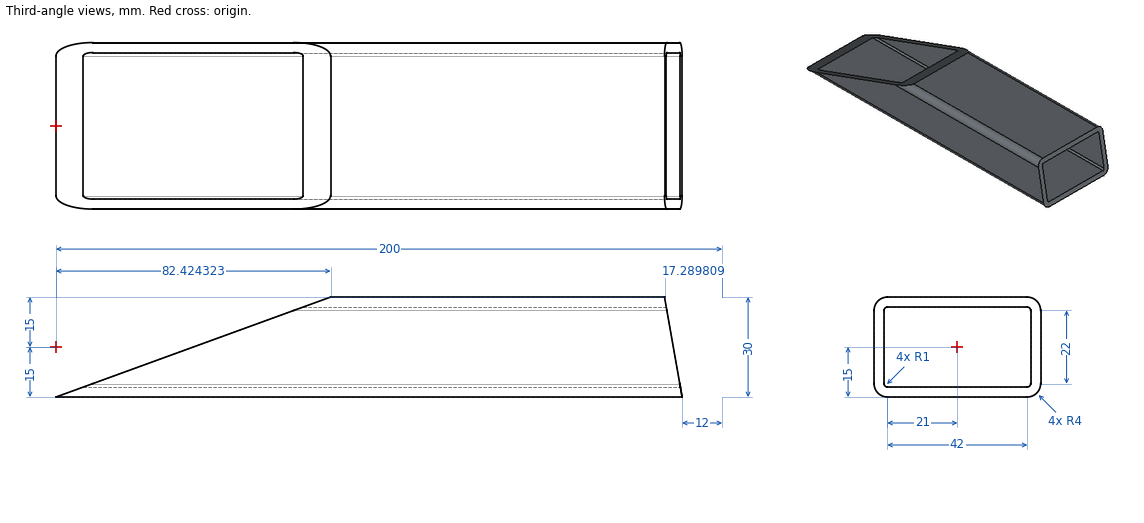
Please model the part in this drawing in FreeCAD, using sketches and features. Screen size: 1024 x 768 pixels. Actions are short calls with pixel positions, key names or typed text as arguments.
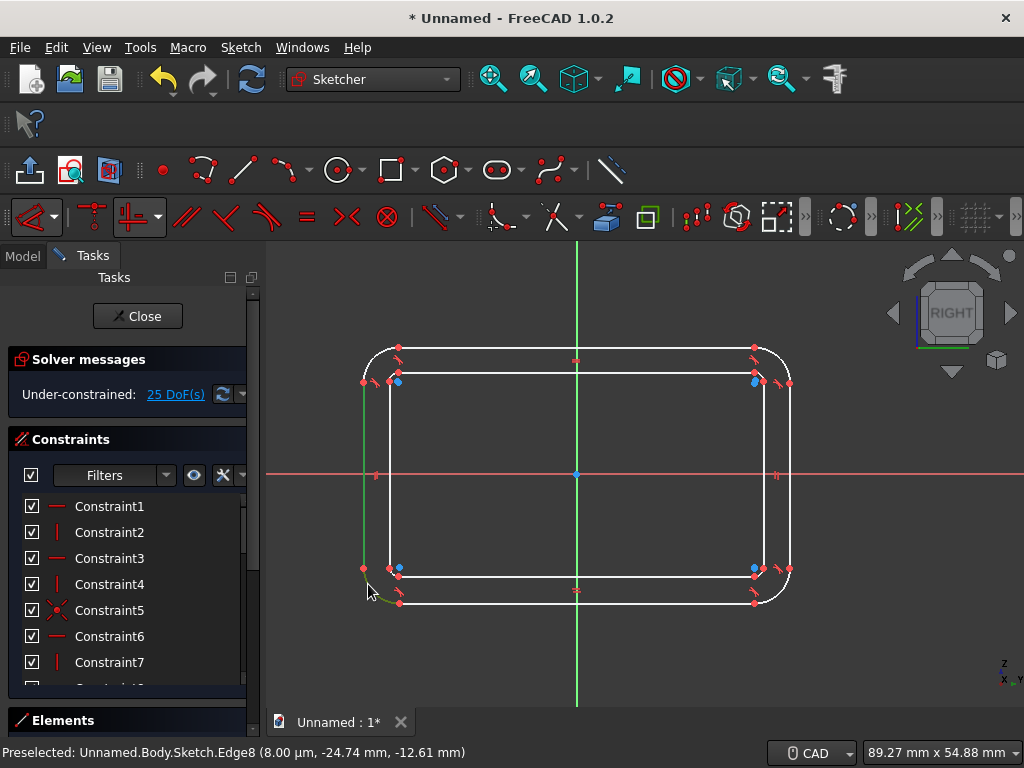
click(268, 218)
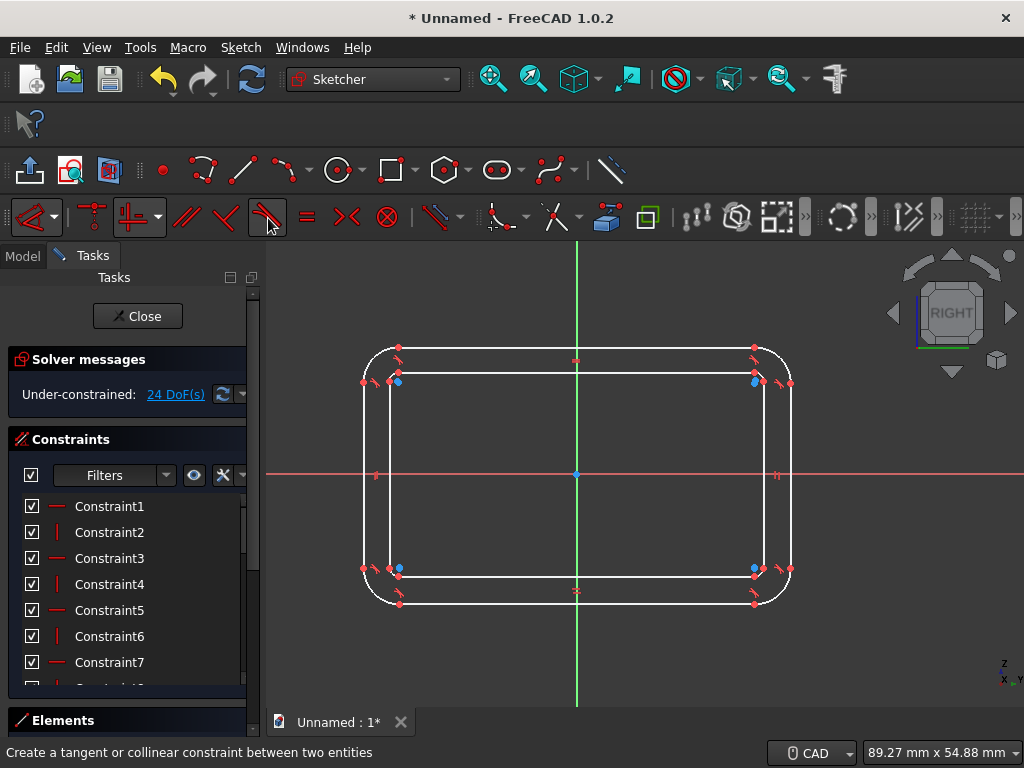
click(648, 577)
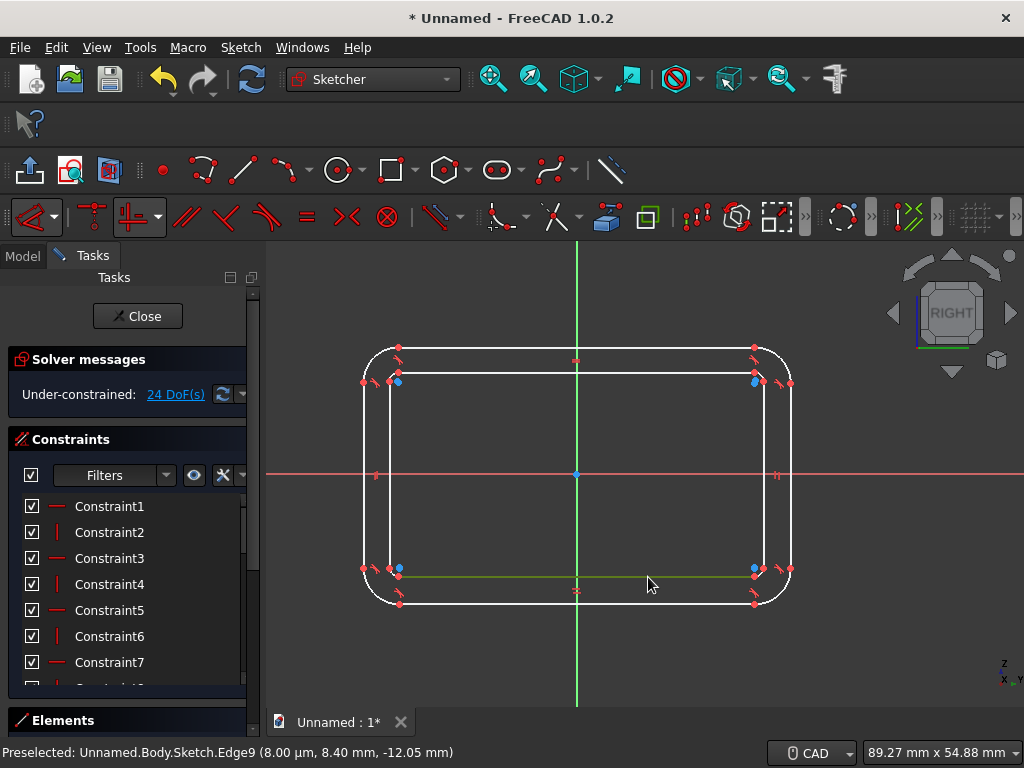
scroll(392, 574, up, 4)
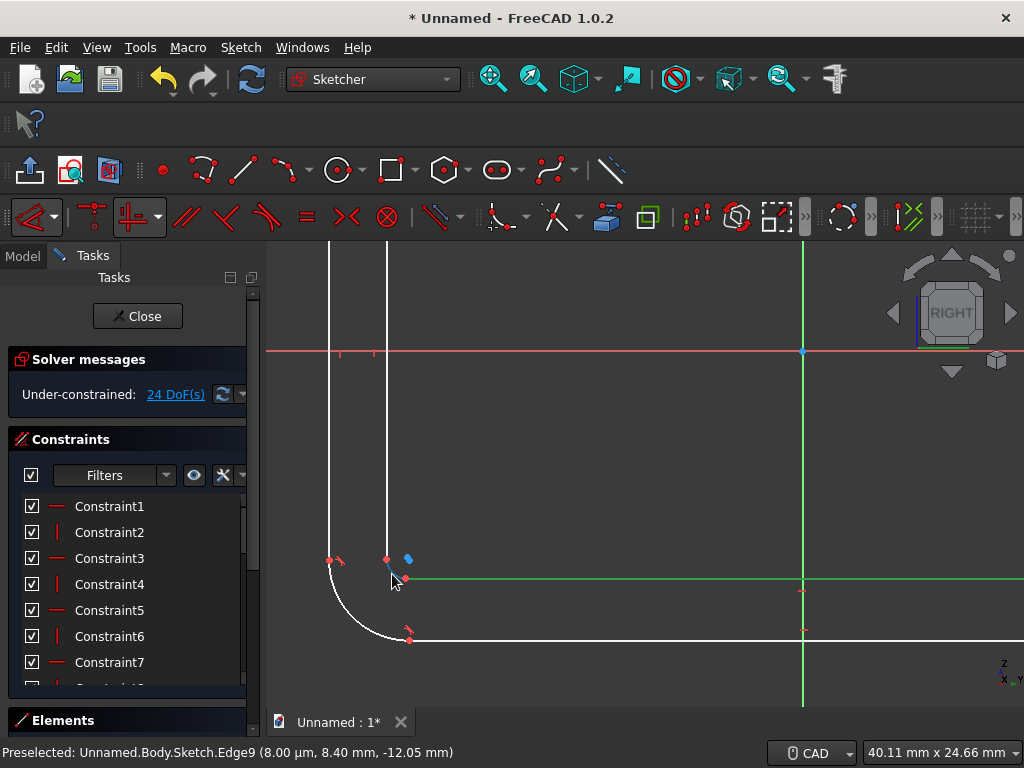
click(393, 573)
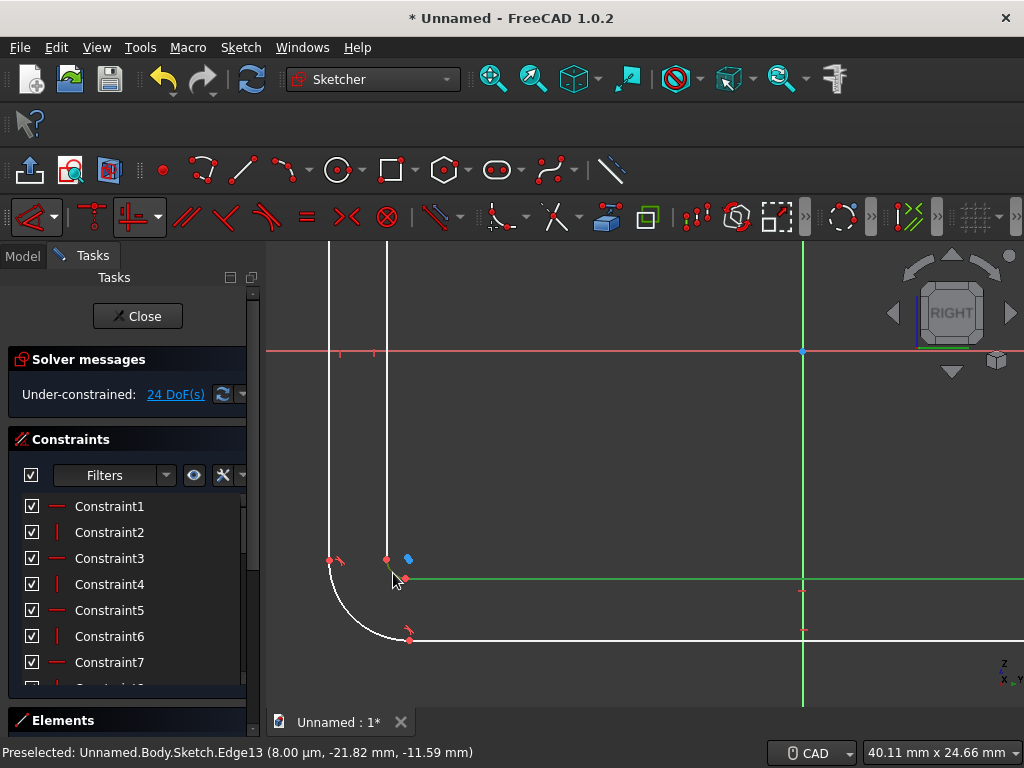
click(268, 218)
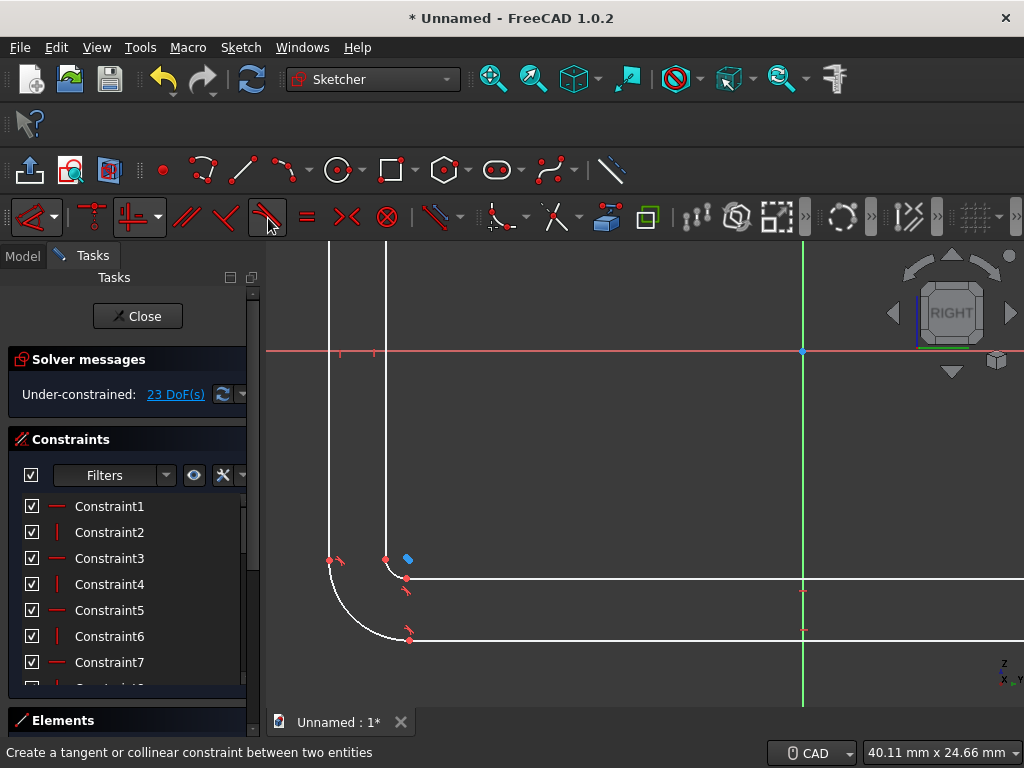
click(645, 579)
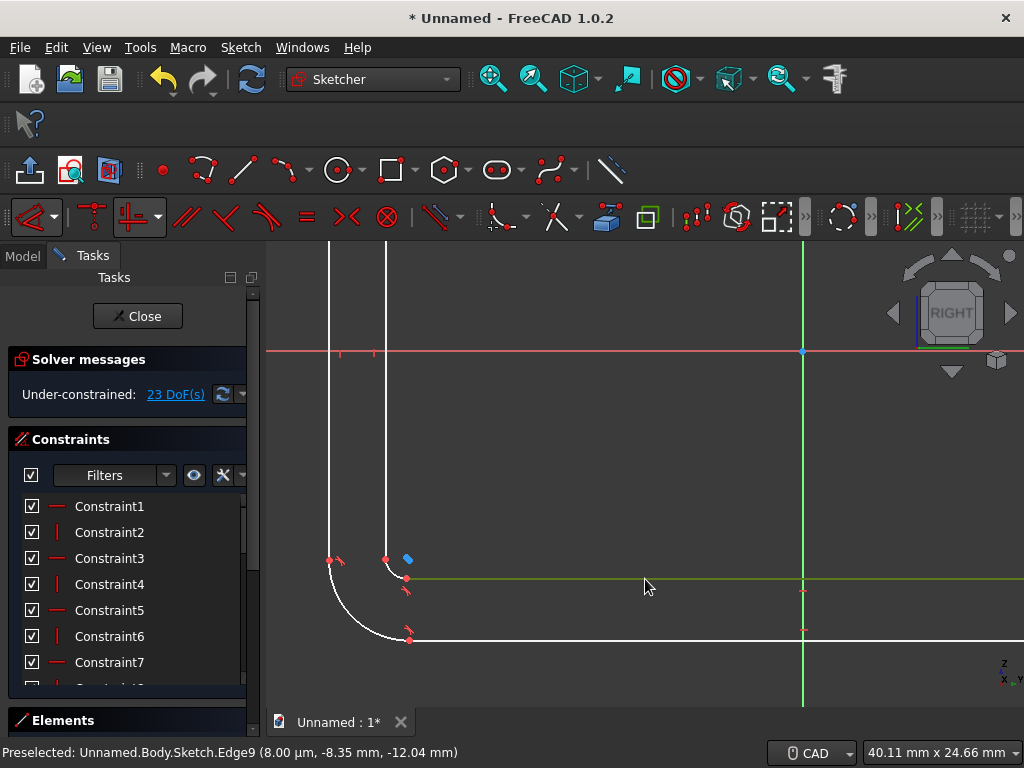
scroll(392, 574, down, 4)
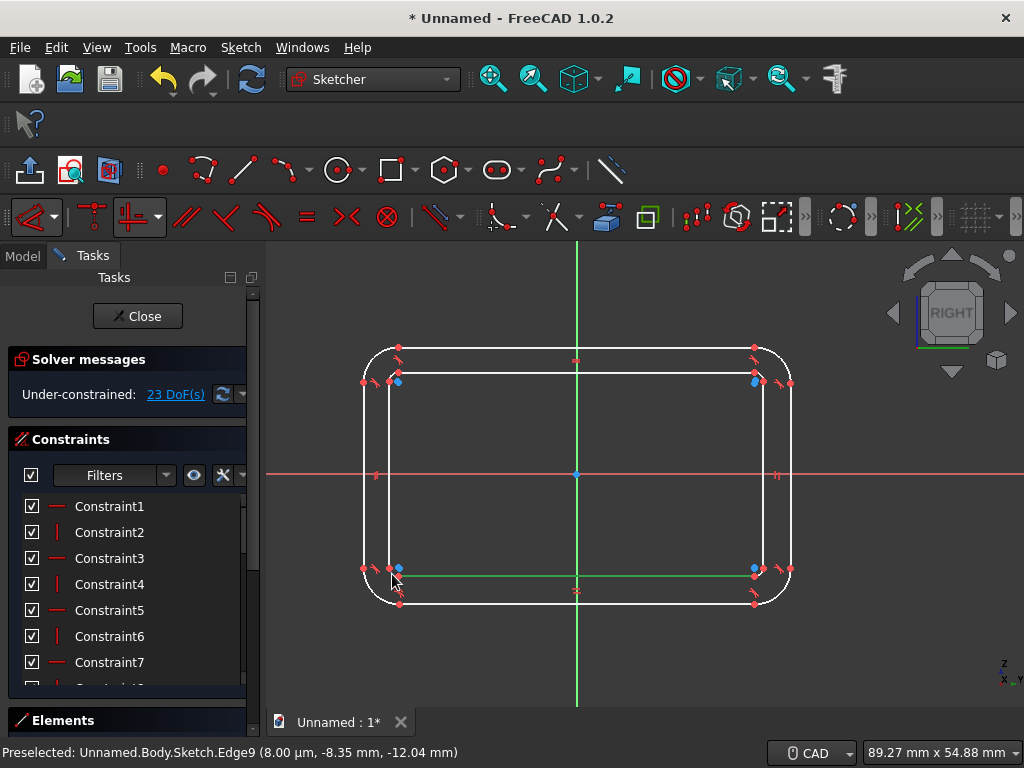
scroll(761, 574, up, 4)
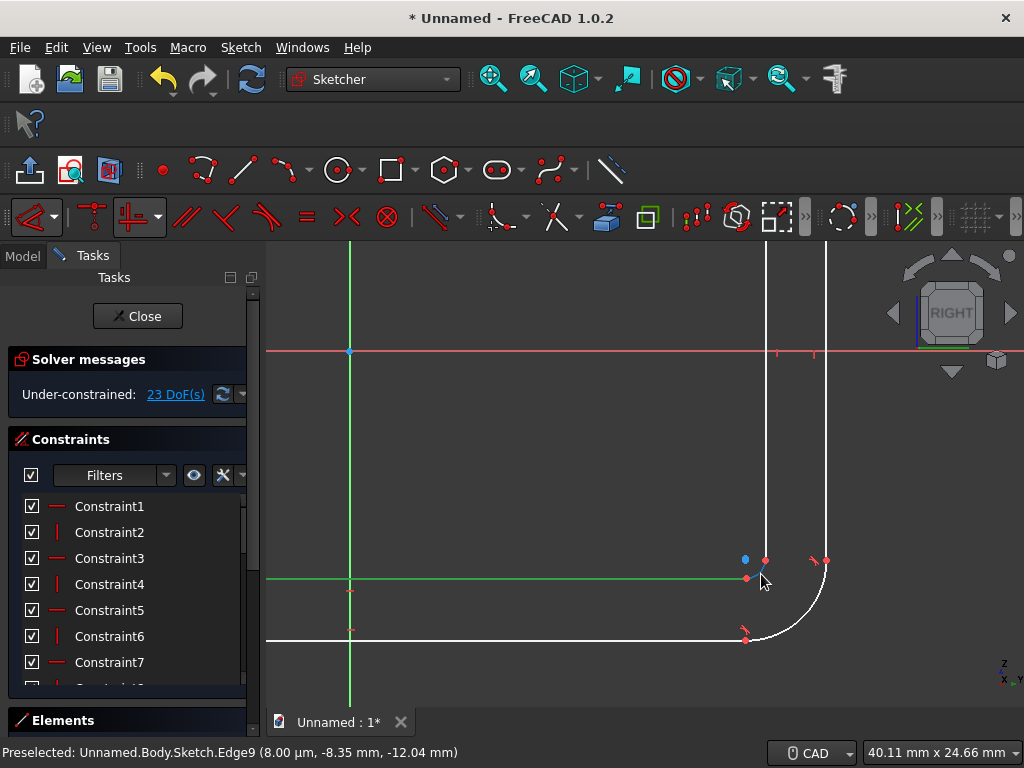
click(760, 573)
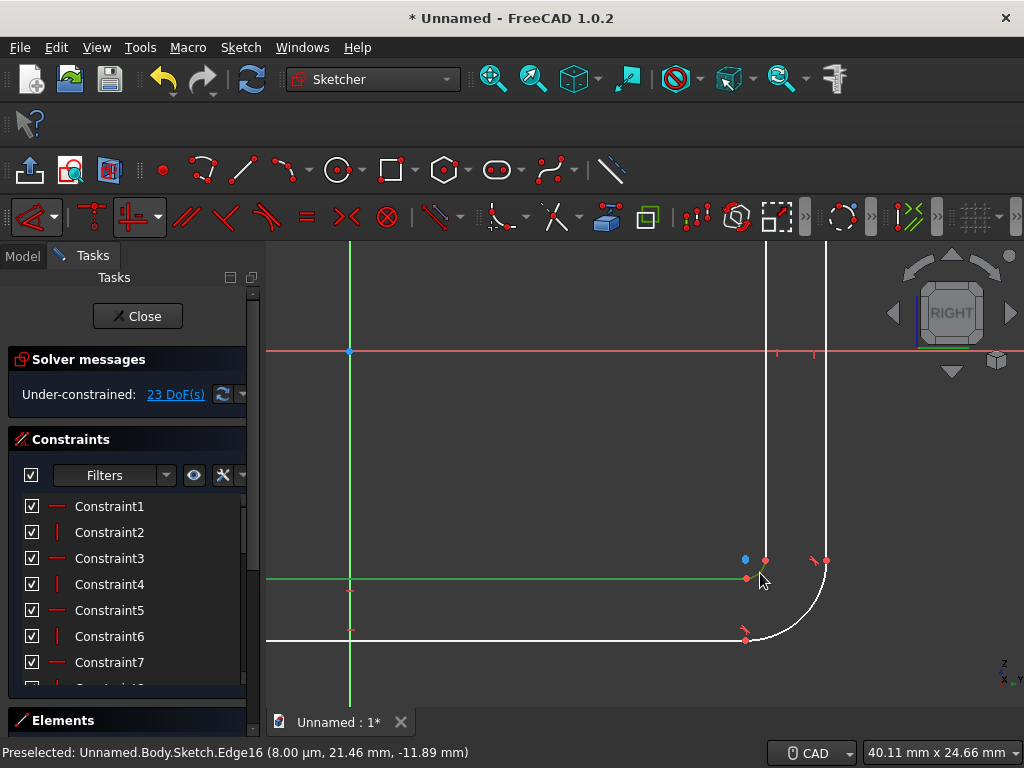
click(268, 218)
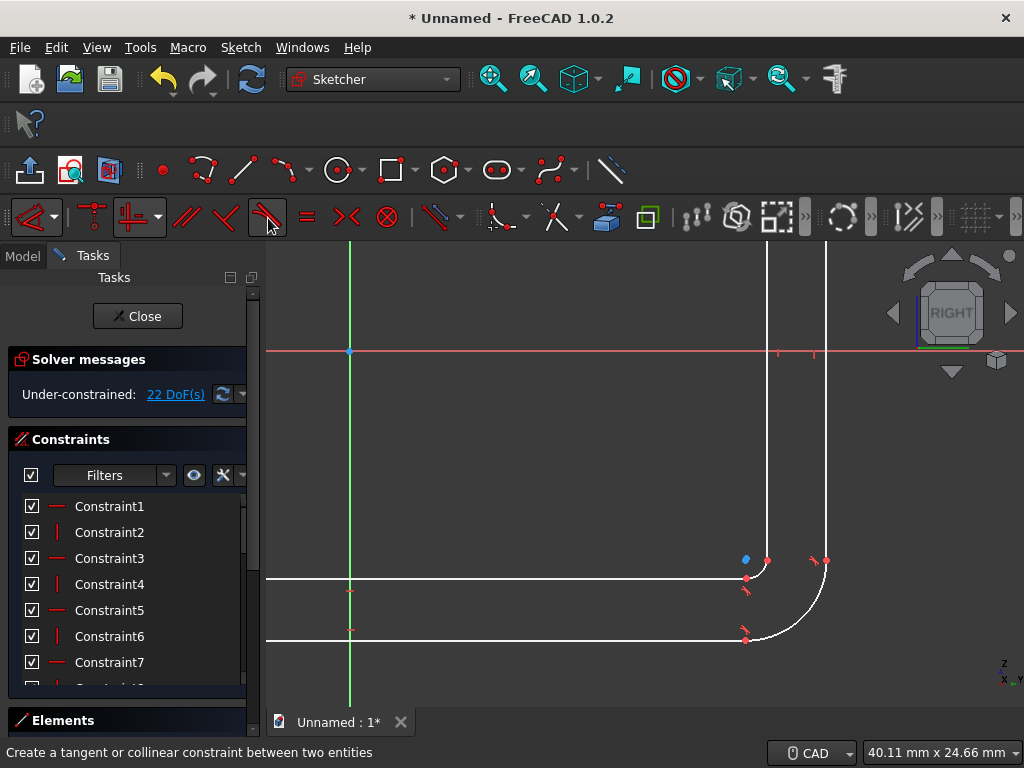
scroll(761, 574, down, 4)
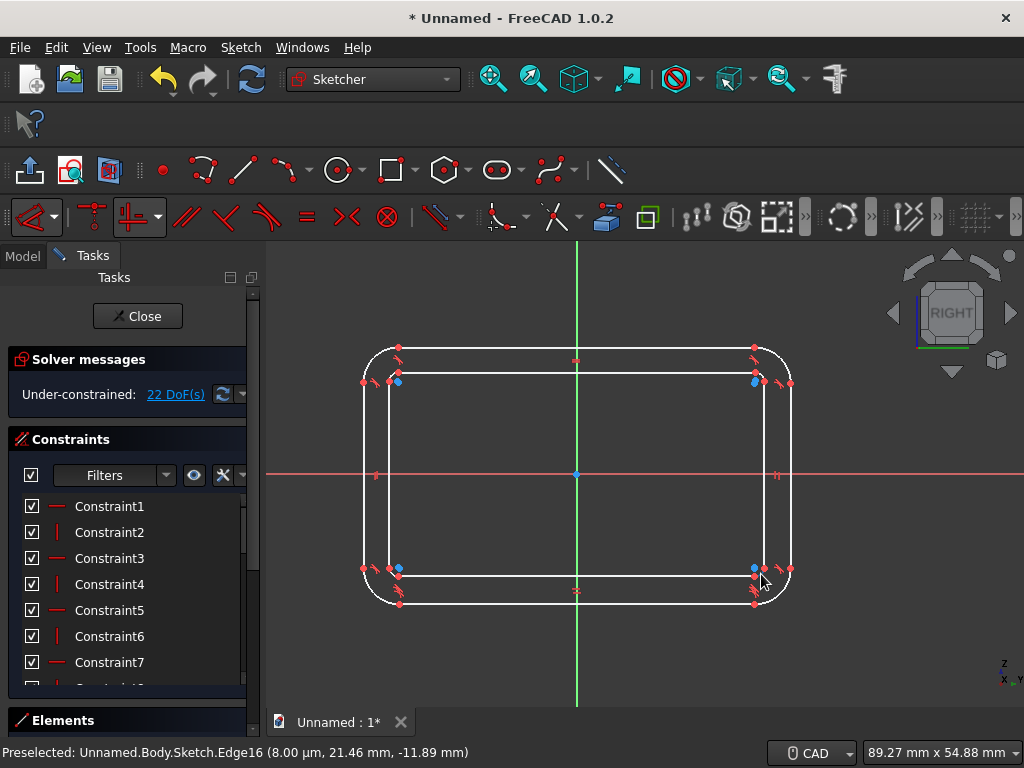
click(389, 512)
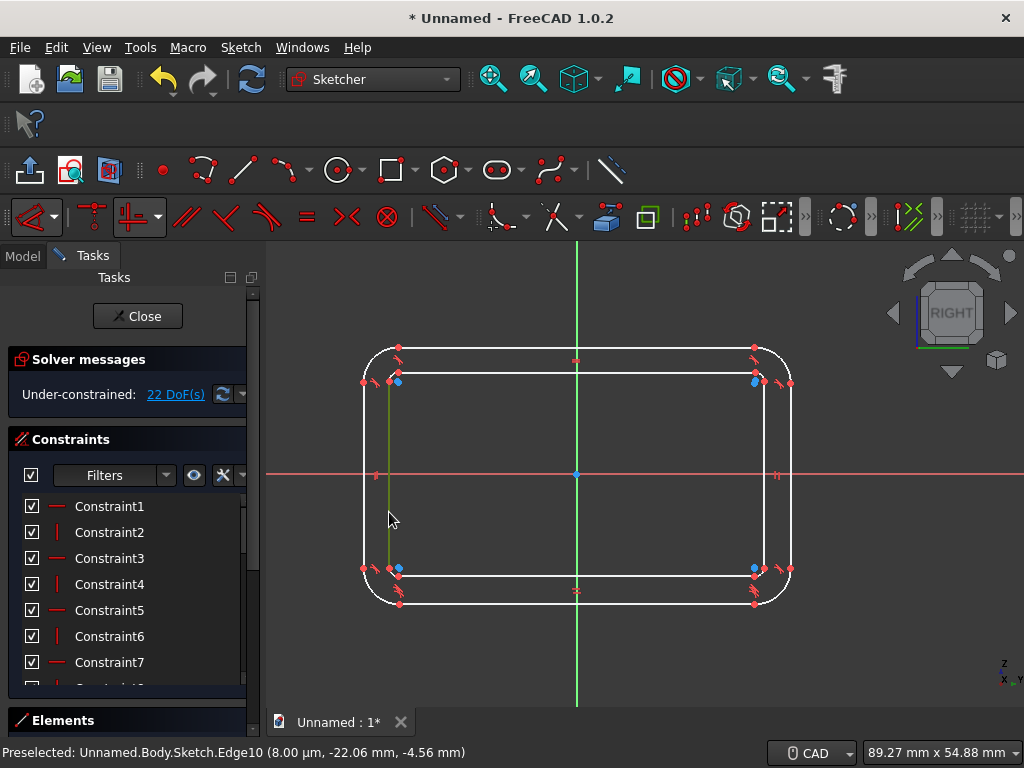
scroll(392, 574, up, 4)